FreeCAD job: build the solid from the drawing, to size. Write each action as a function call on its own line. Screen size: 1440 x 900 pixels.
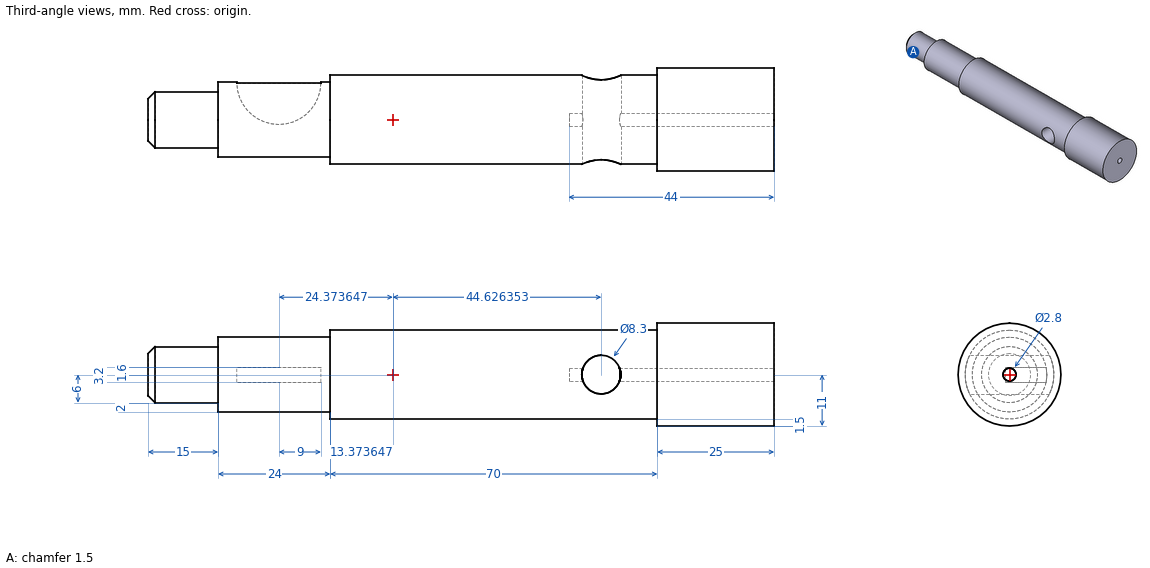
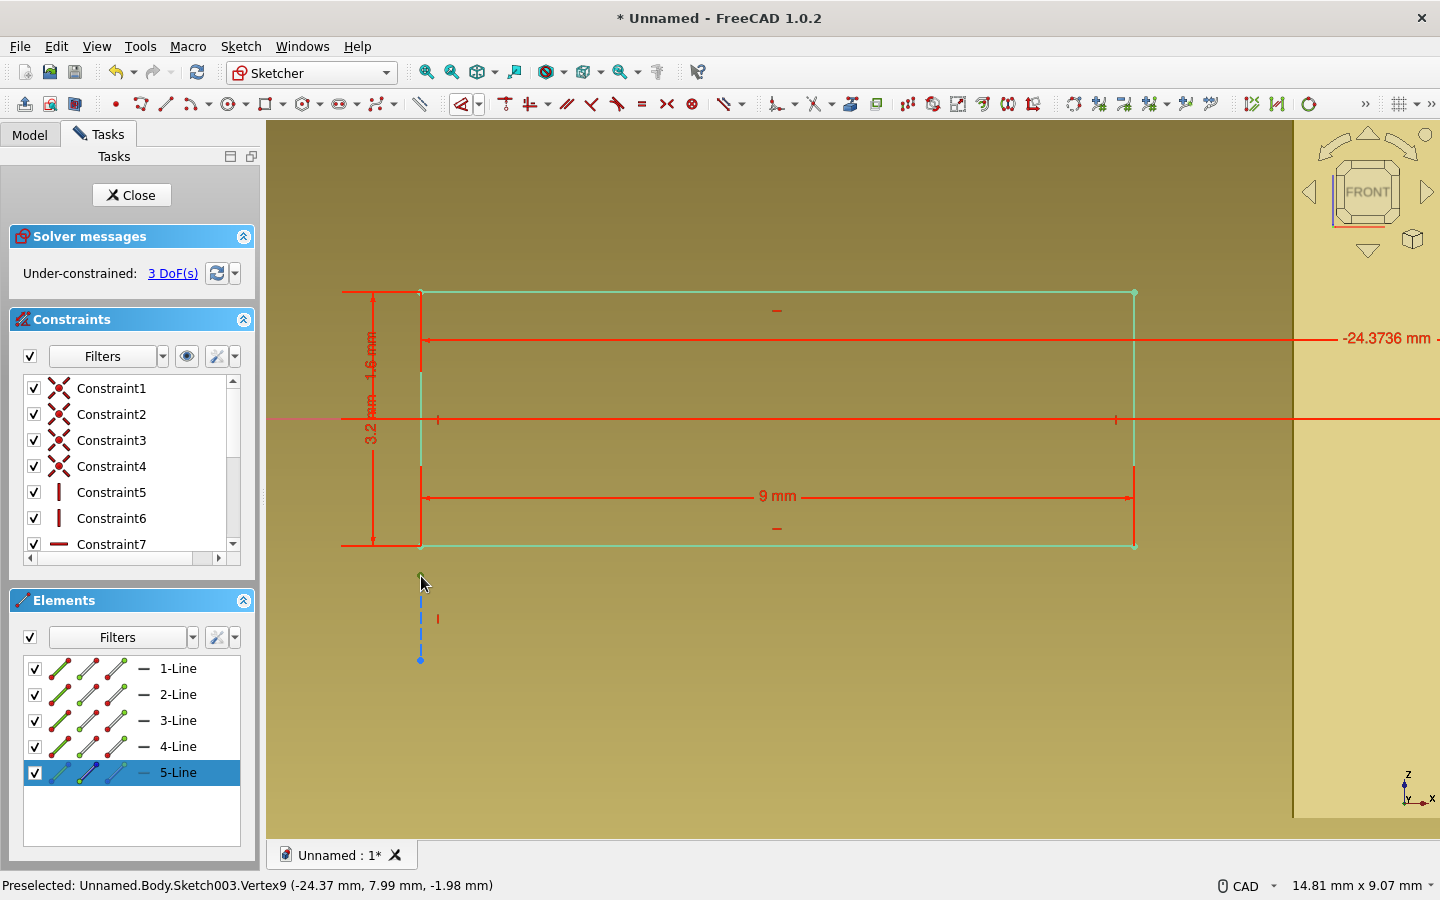
click(478, 104)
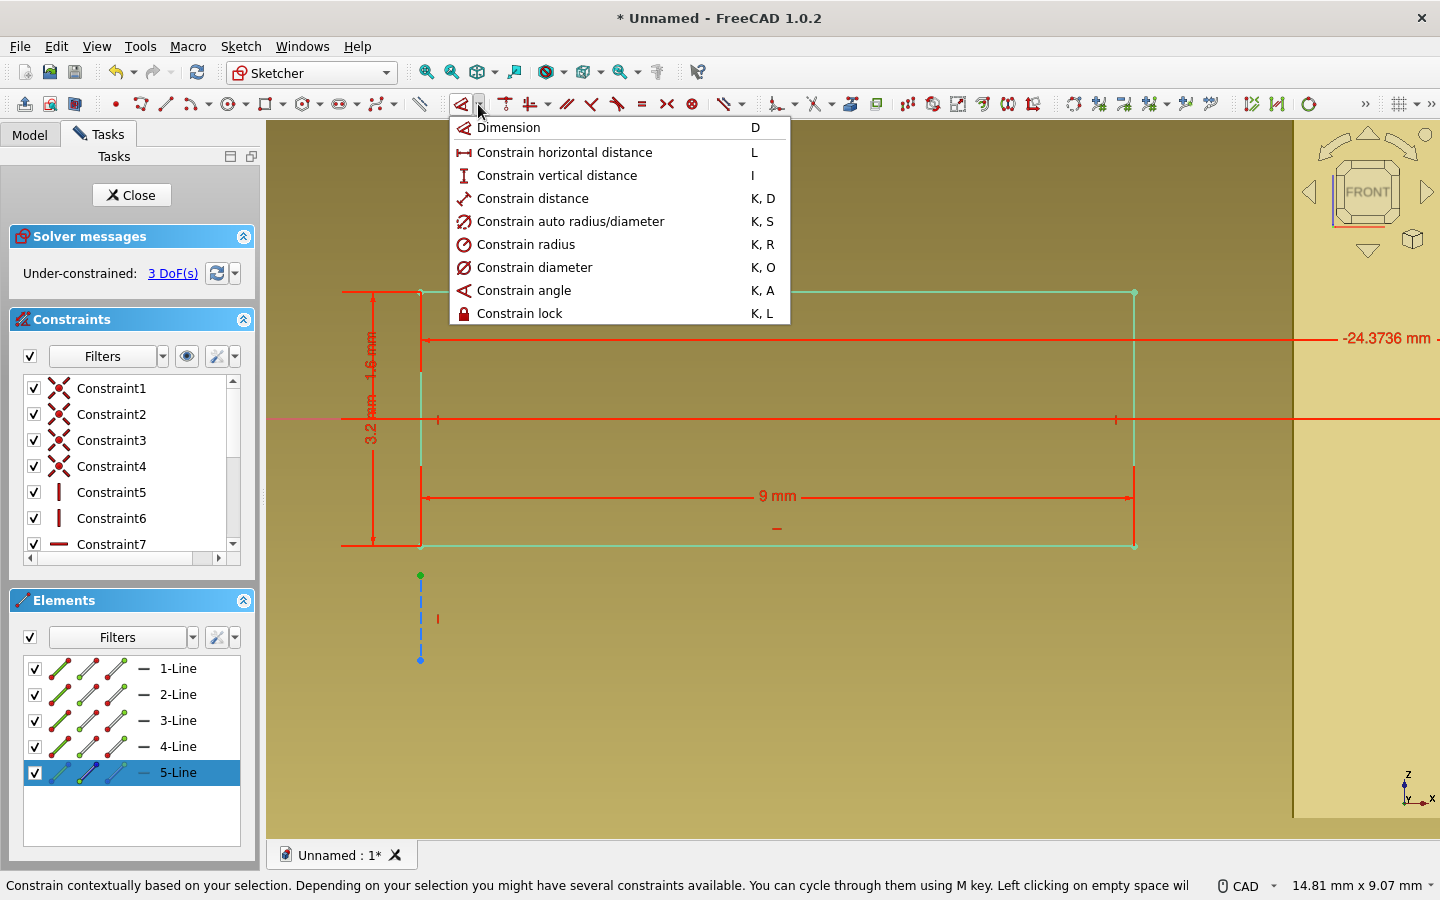
click(620, 152)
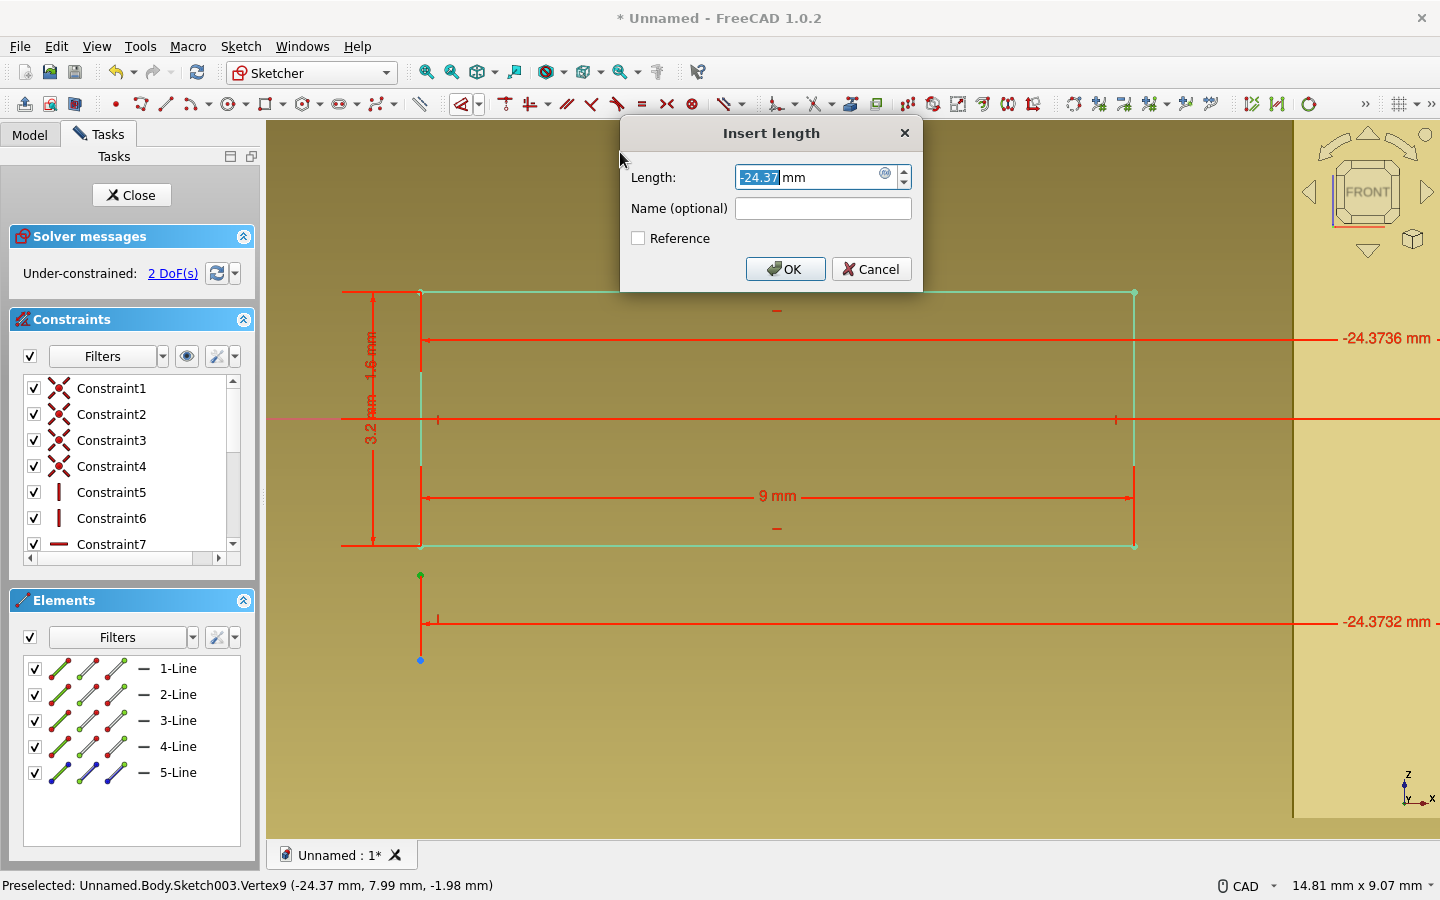
text(-24.373647)
key(Return)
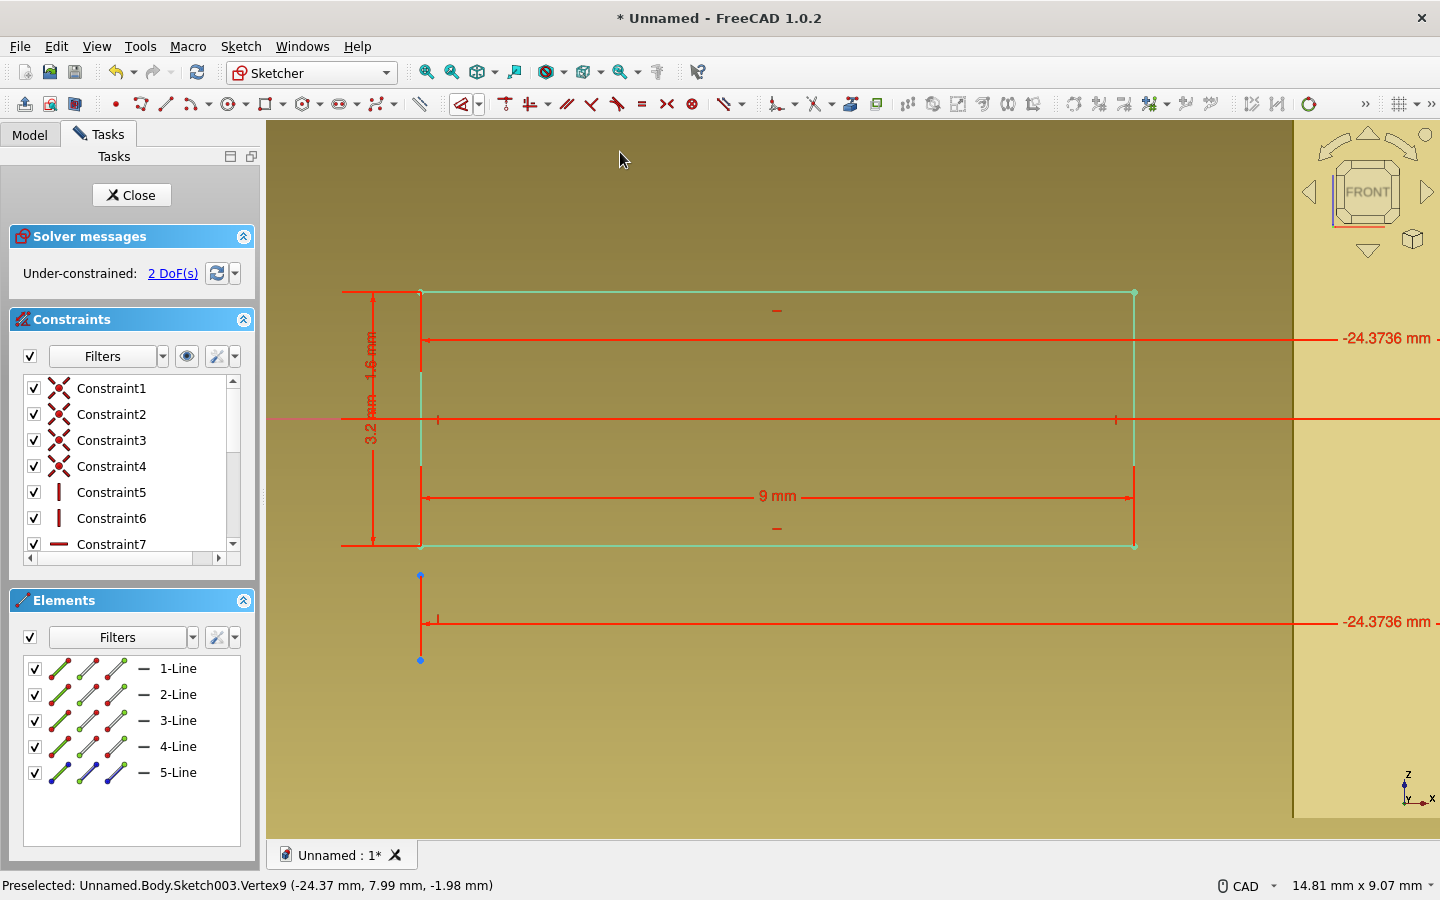
click(132, 195)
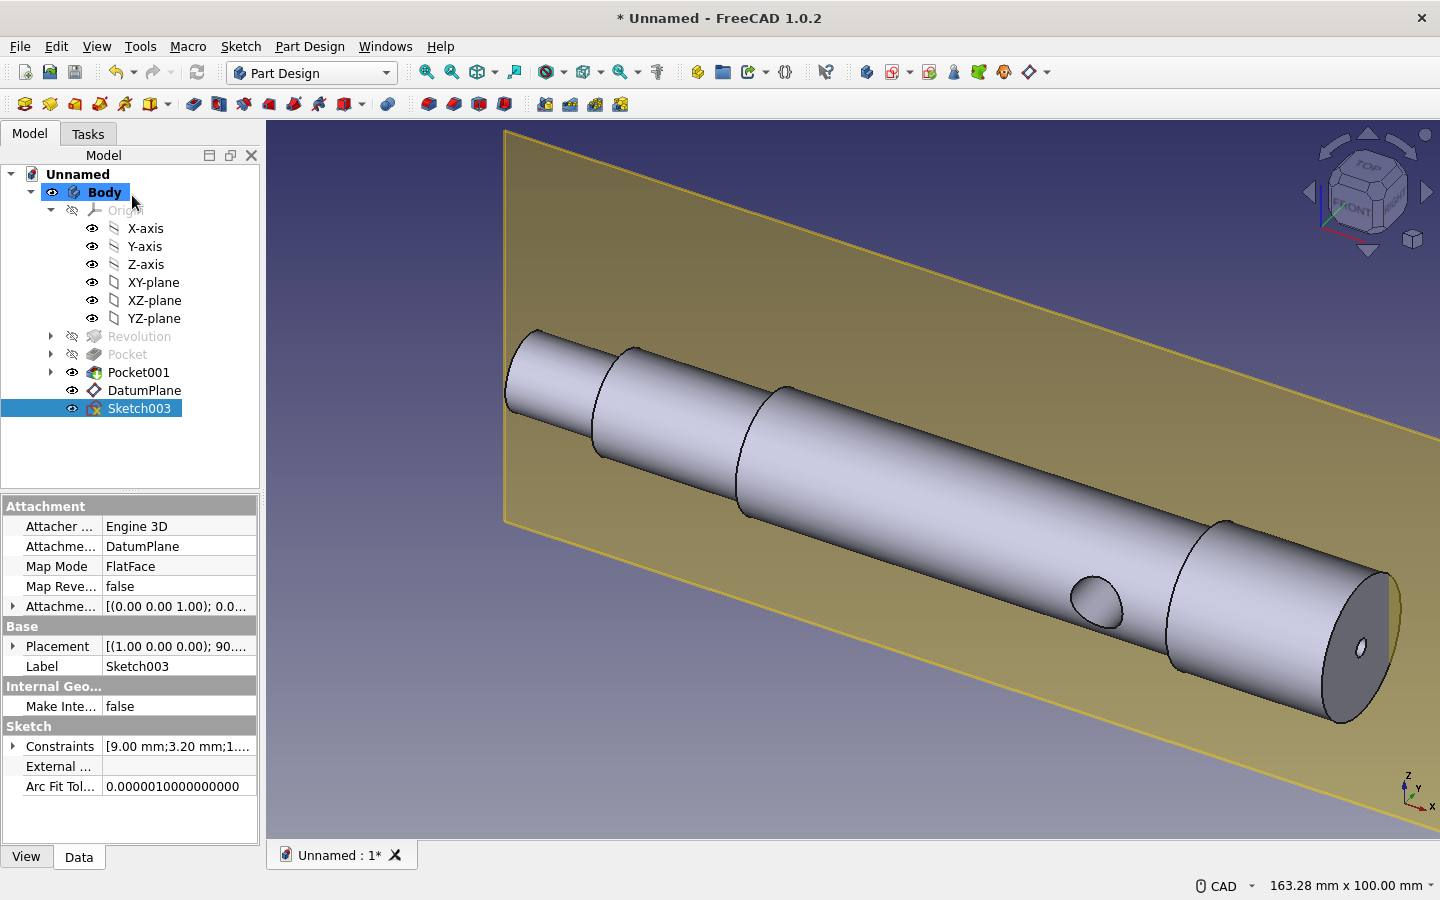
click(244, 104)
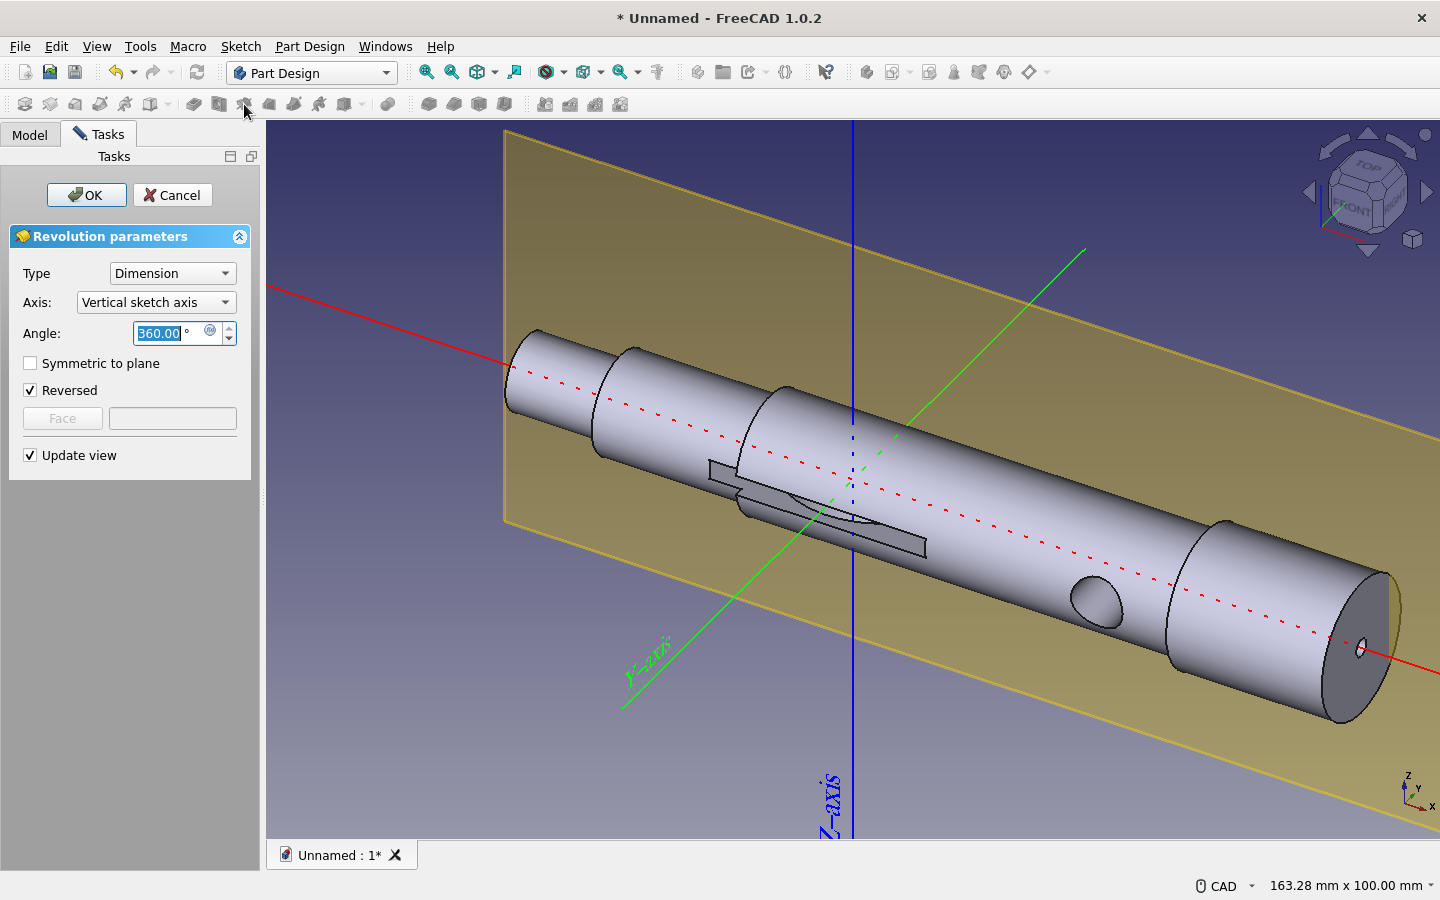
click(157, 302)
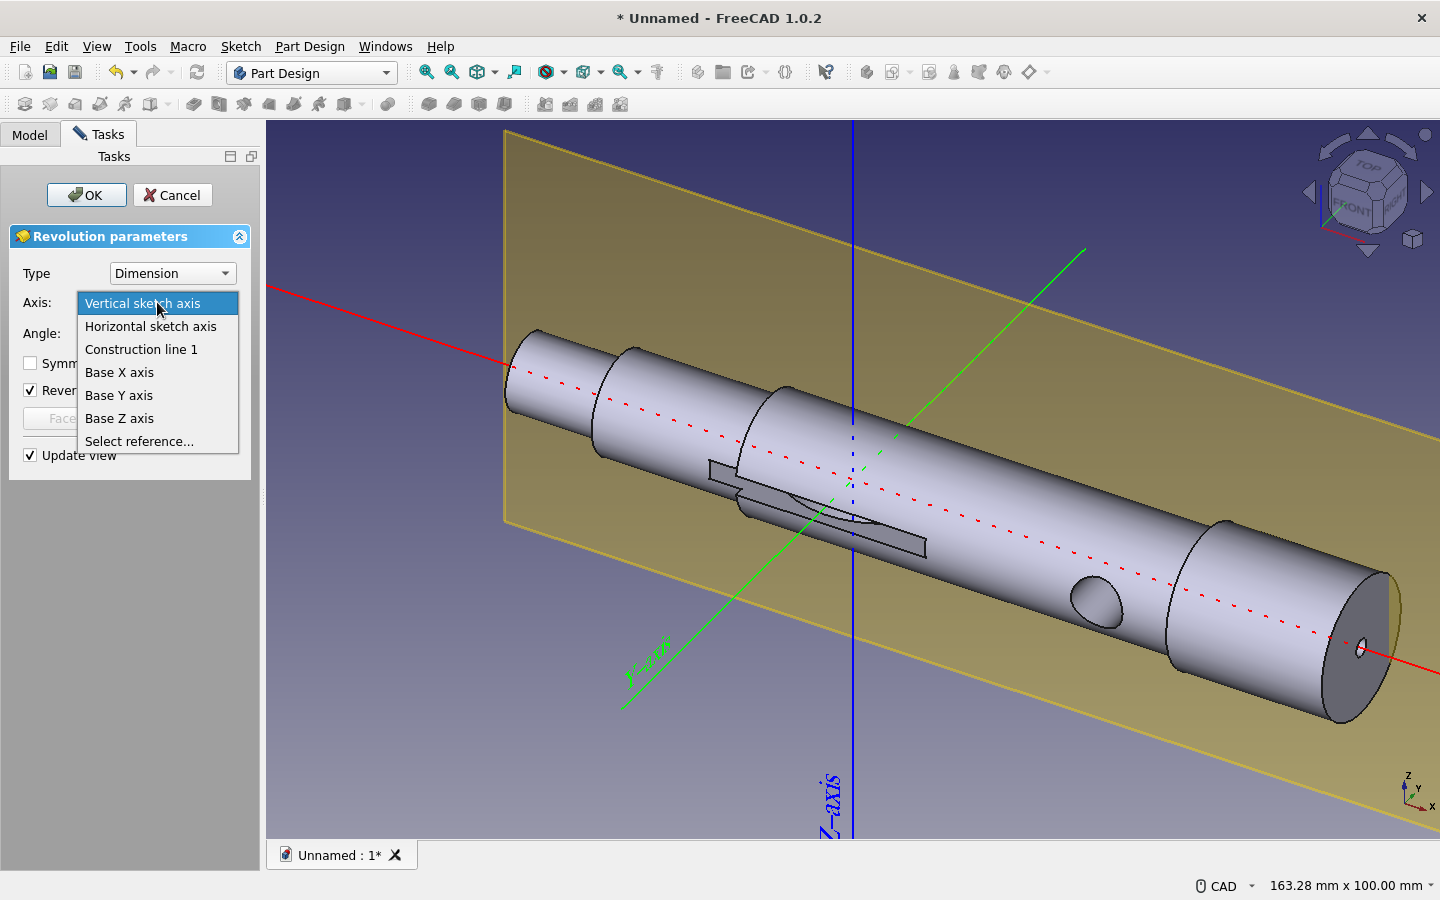
click(156, 350)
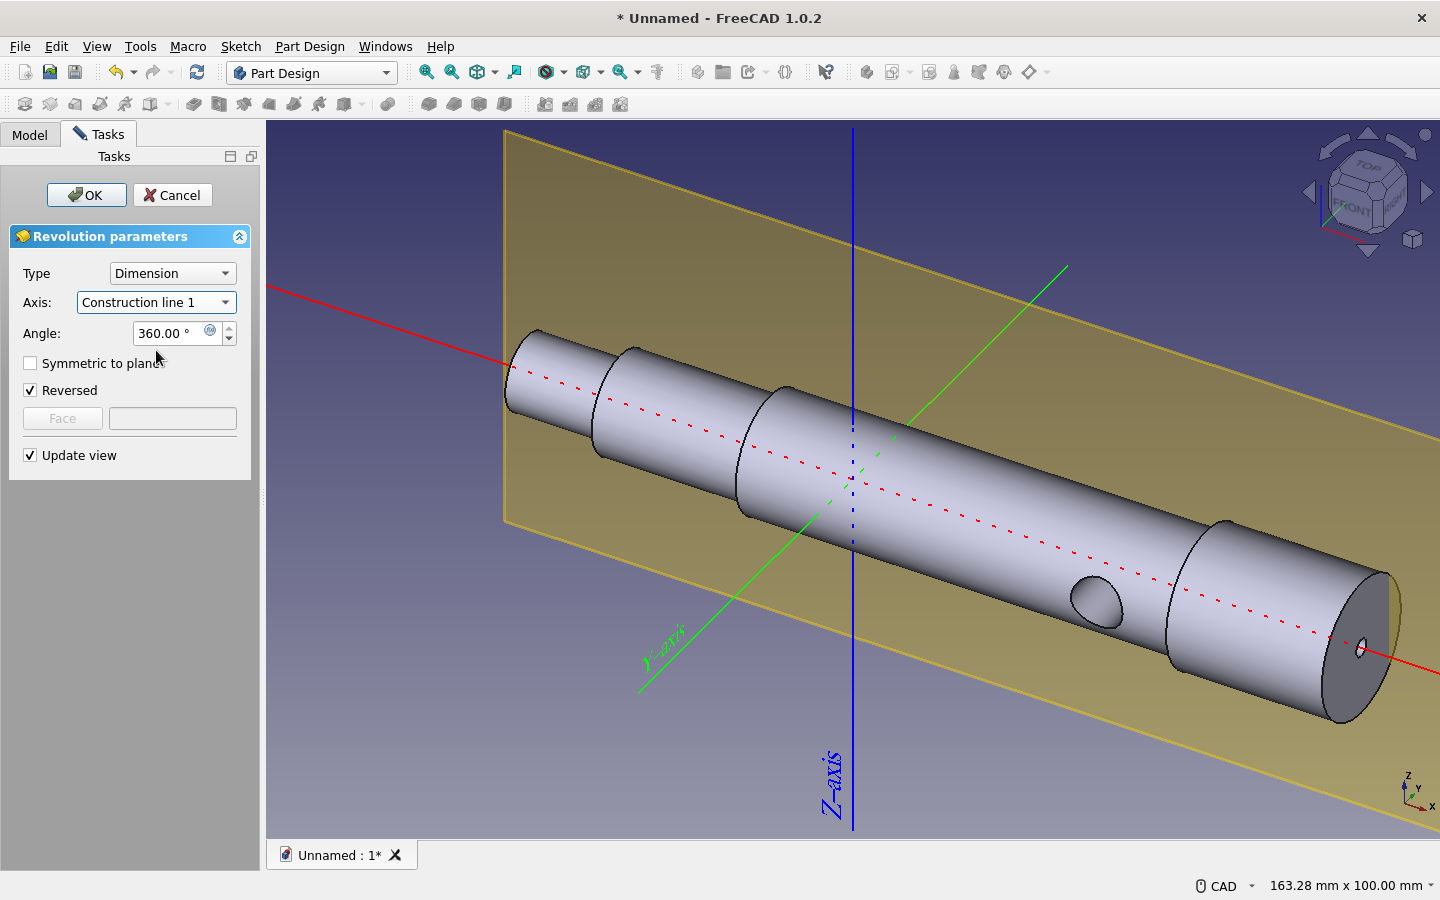
click(87, 195)